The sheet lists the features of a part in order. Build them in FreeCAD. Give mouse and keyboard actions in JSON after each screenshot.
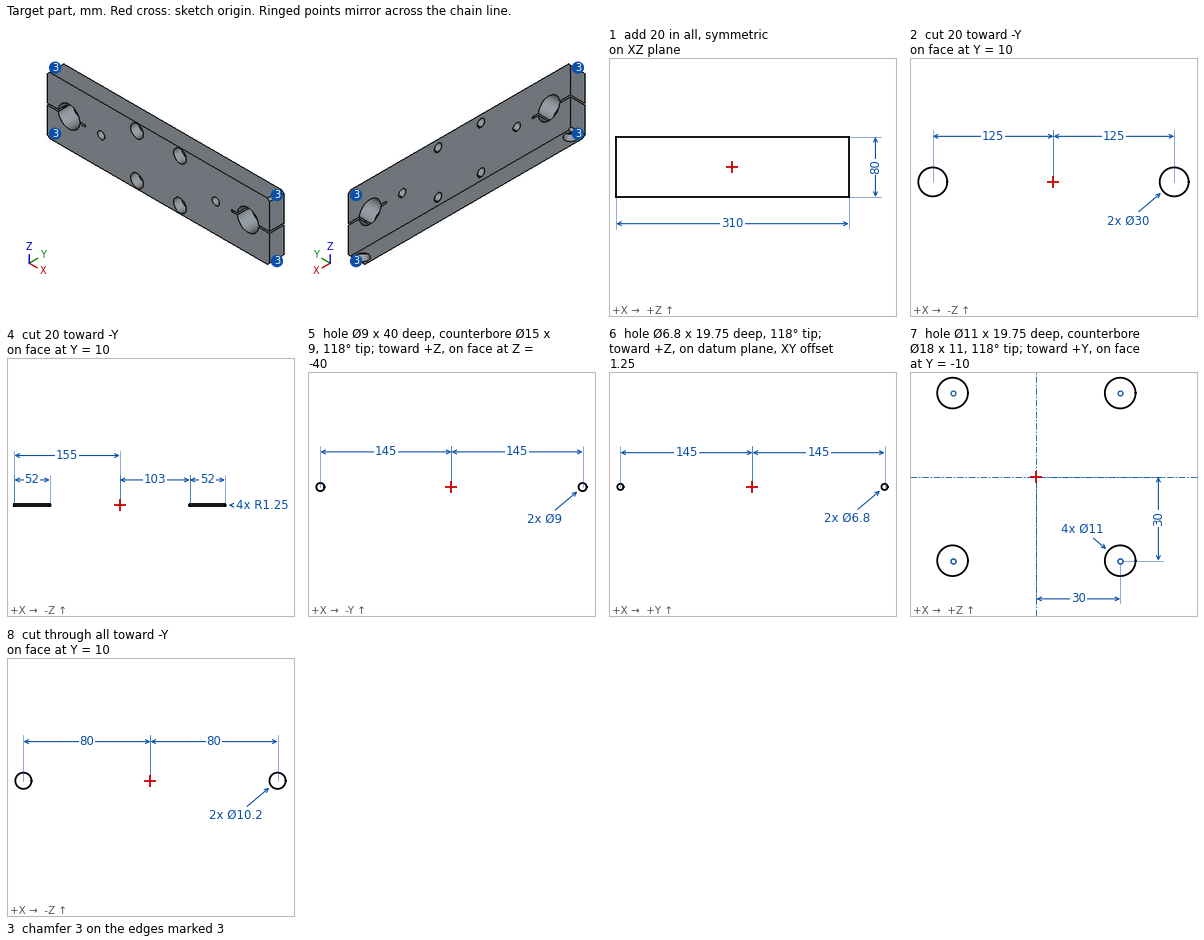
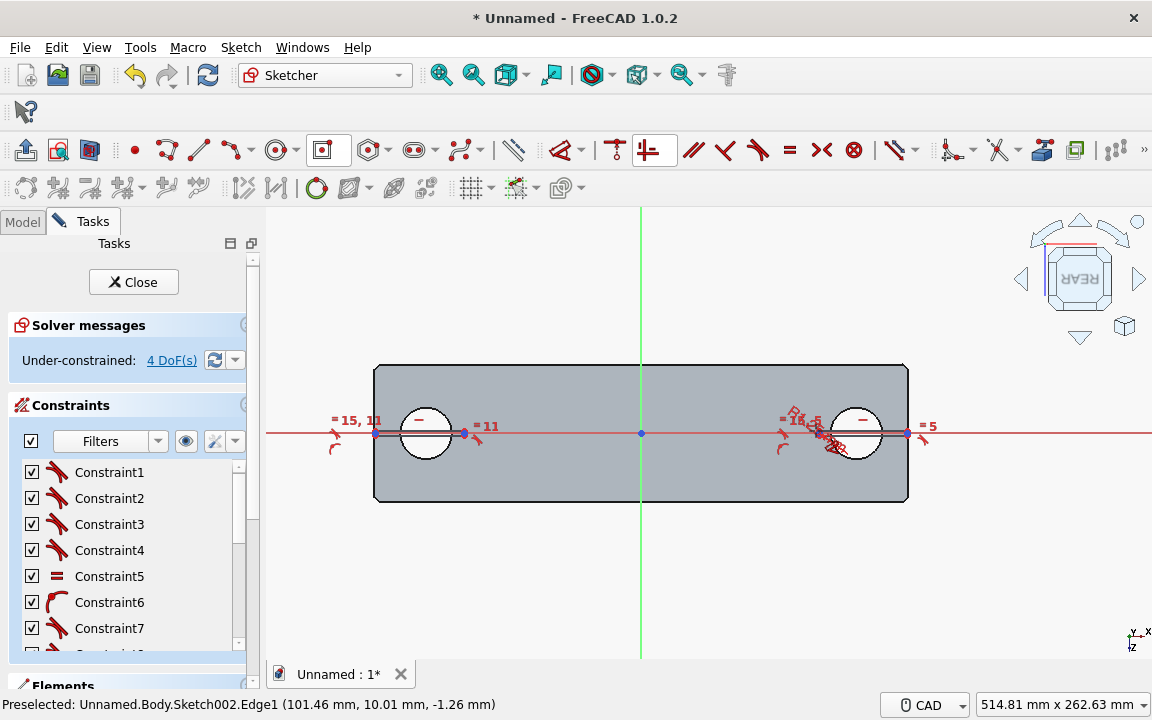
{"action": "scroll", "coordinate": [846, 431], "scroll_direction": "up", "scroll_amount": 10}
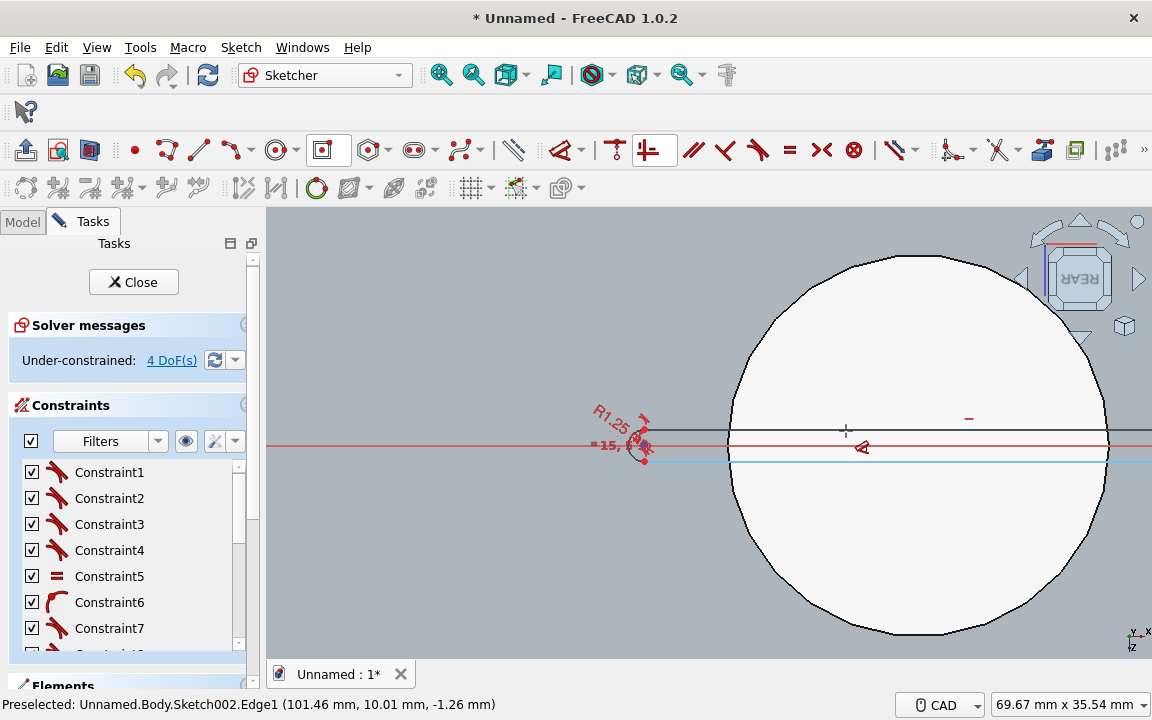
{"action": "left_click", "coordinate": [840, 430]}
{"action": "left_click", "coordinate": [816, 396]}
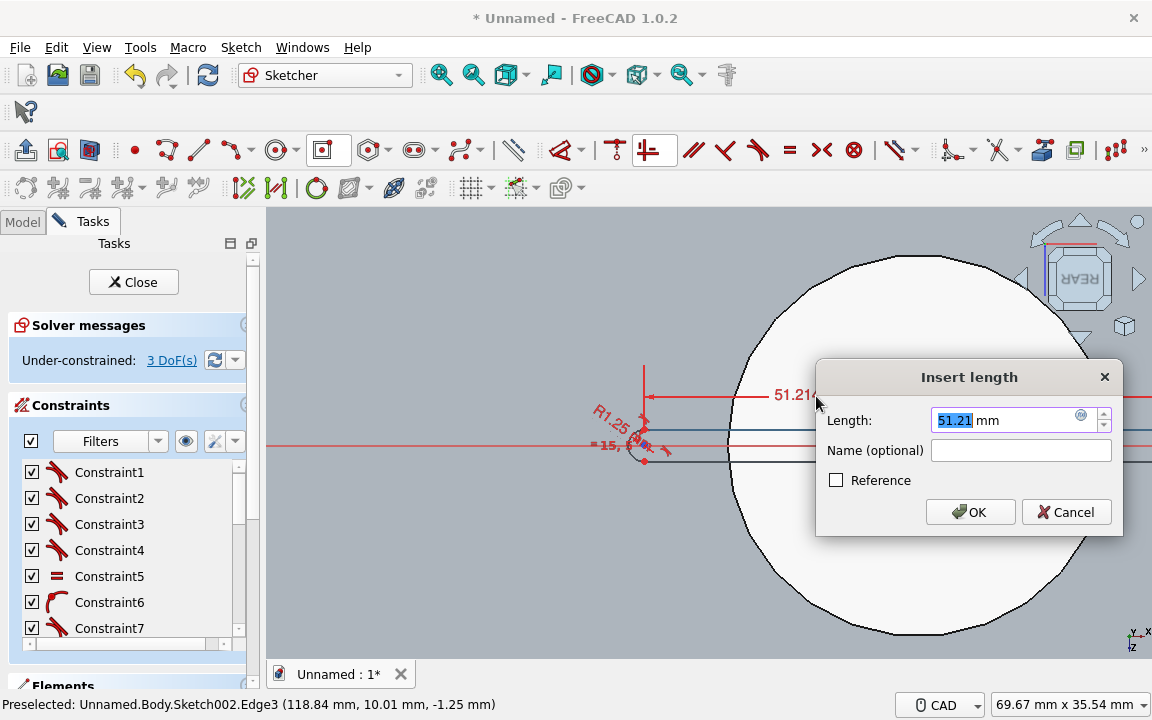
{"action": "type", "text": "52"}
{"action": "key", "text": "Return"}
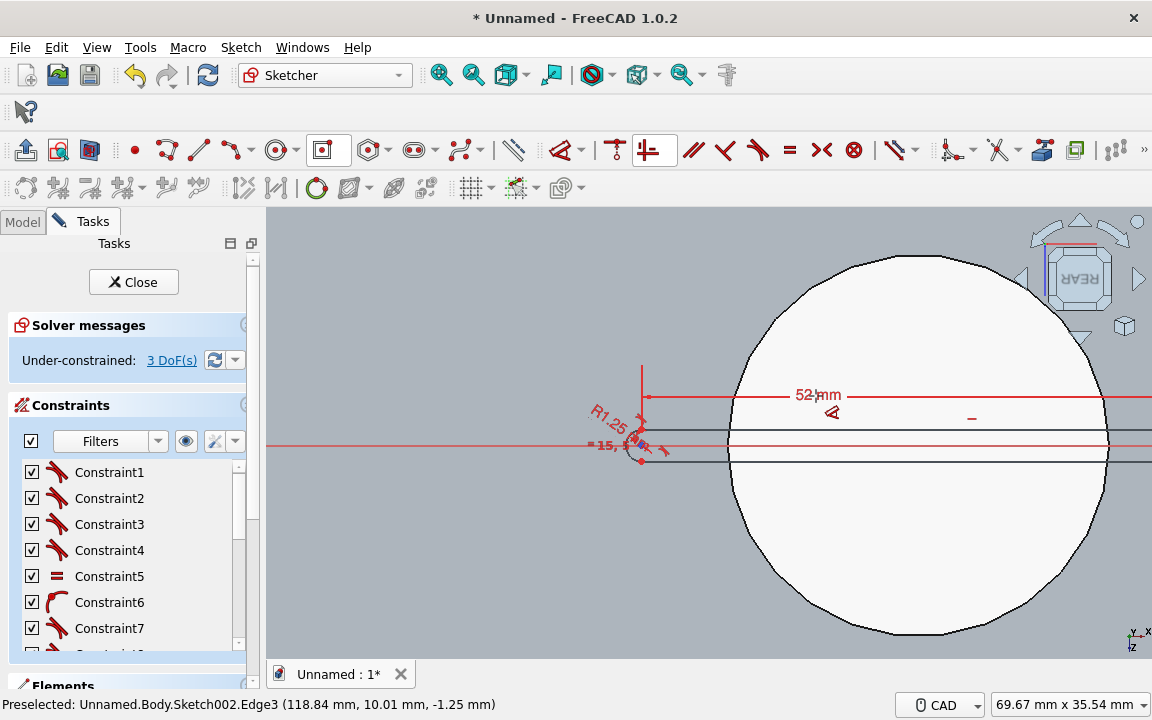
{"action": "scroll", "coordinate": [846, 431], "scroll_direction": "down", "scroll_amount": 10}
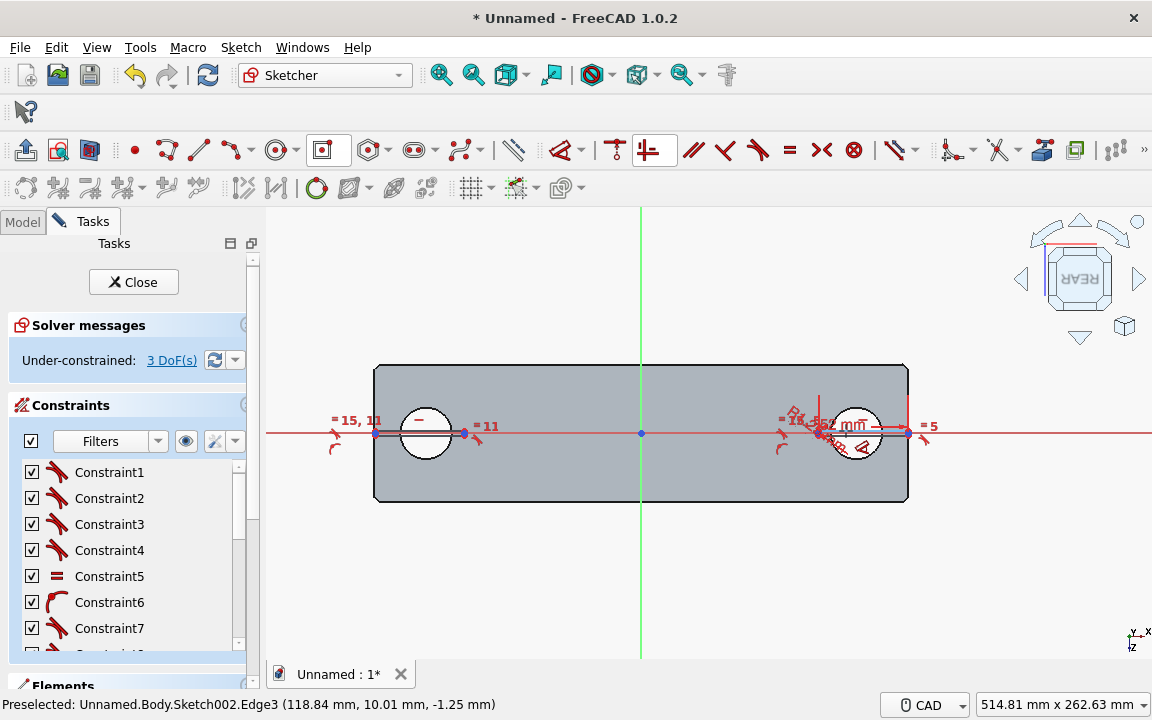
{"action": "scroll", "coordinate": [402, 431], "scroll_direction": "up", "scroll_amount": 10}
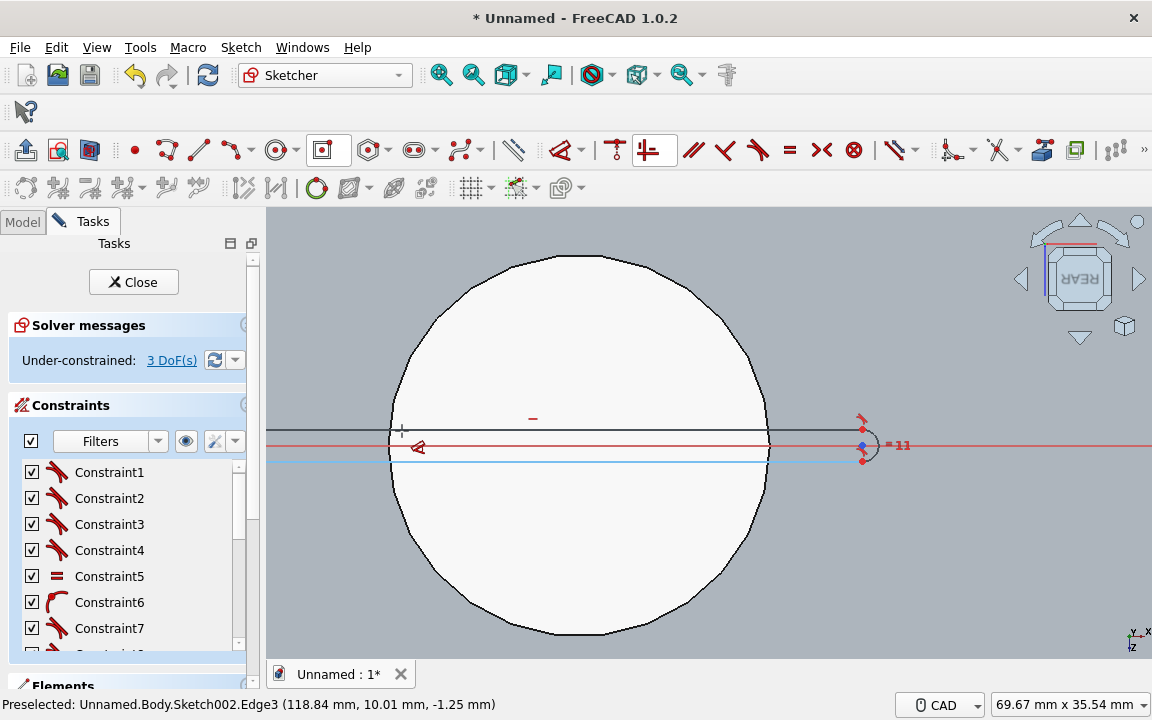
{"action": "left_click", "coordinate": [402, 430]}
{"action": "left_click", "coordinate": [578, 396]}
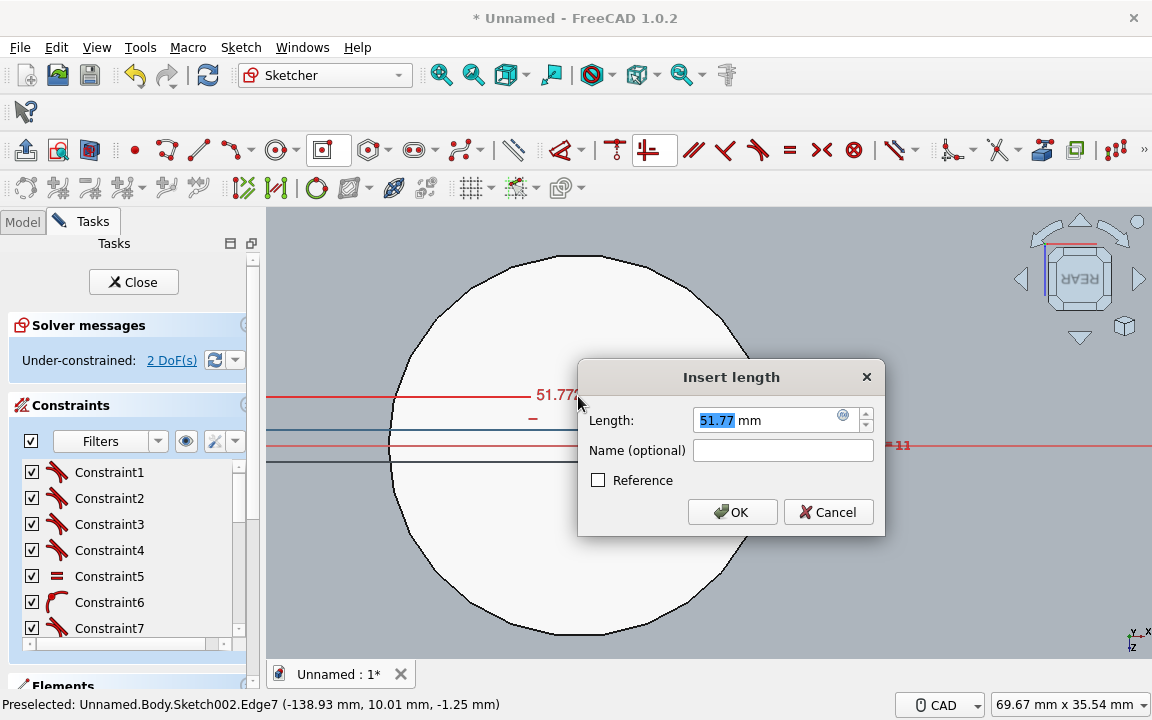
{"action": "type", "text": "52"}
{"action": "key", "text": "Return"}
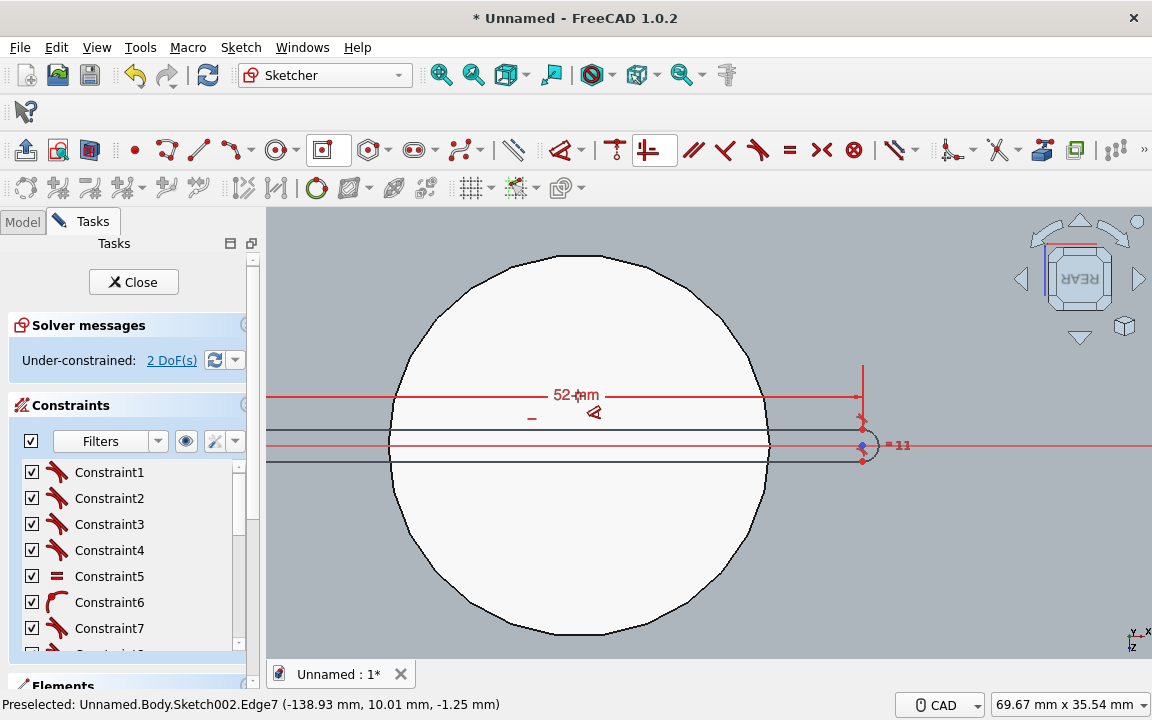
{"action": "scroll", "coordinate": [401, 431], "scroll_direction": "down", "scroll_amount": 10}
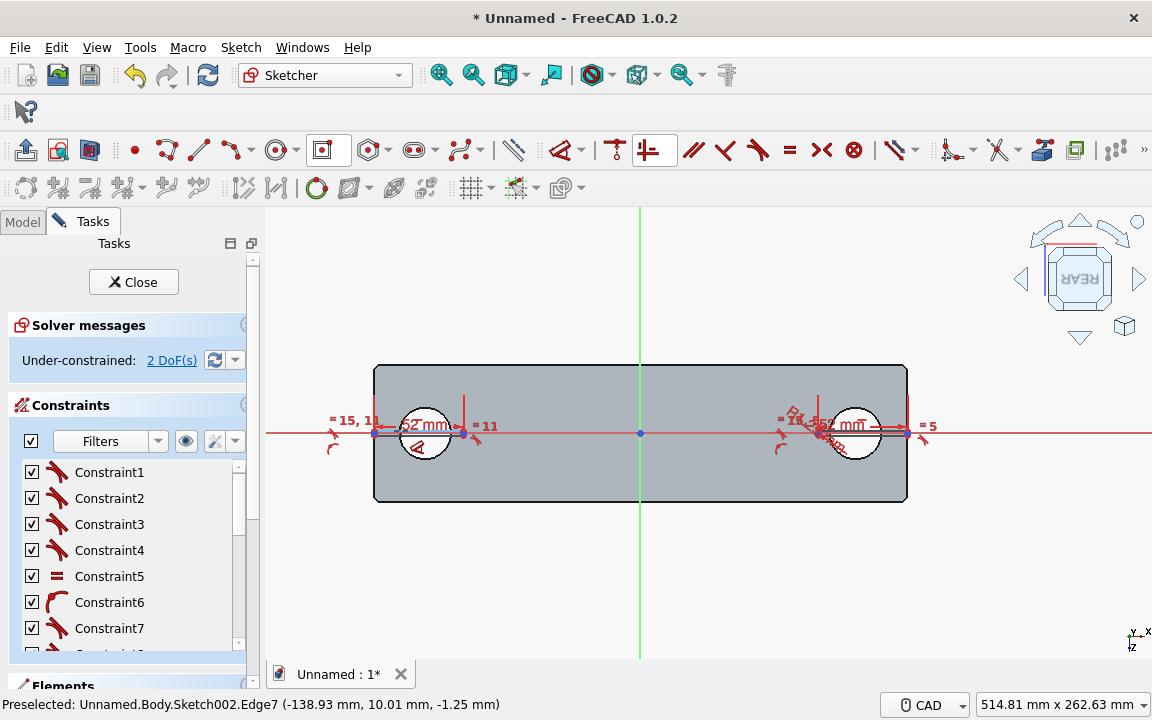
{"action": "scroll", "coordinate": [818, 431], "scroll_direction": "up", "scroll_amount": 9}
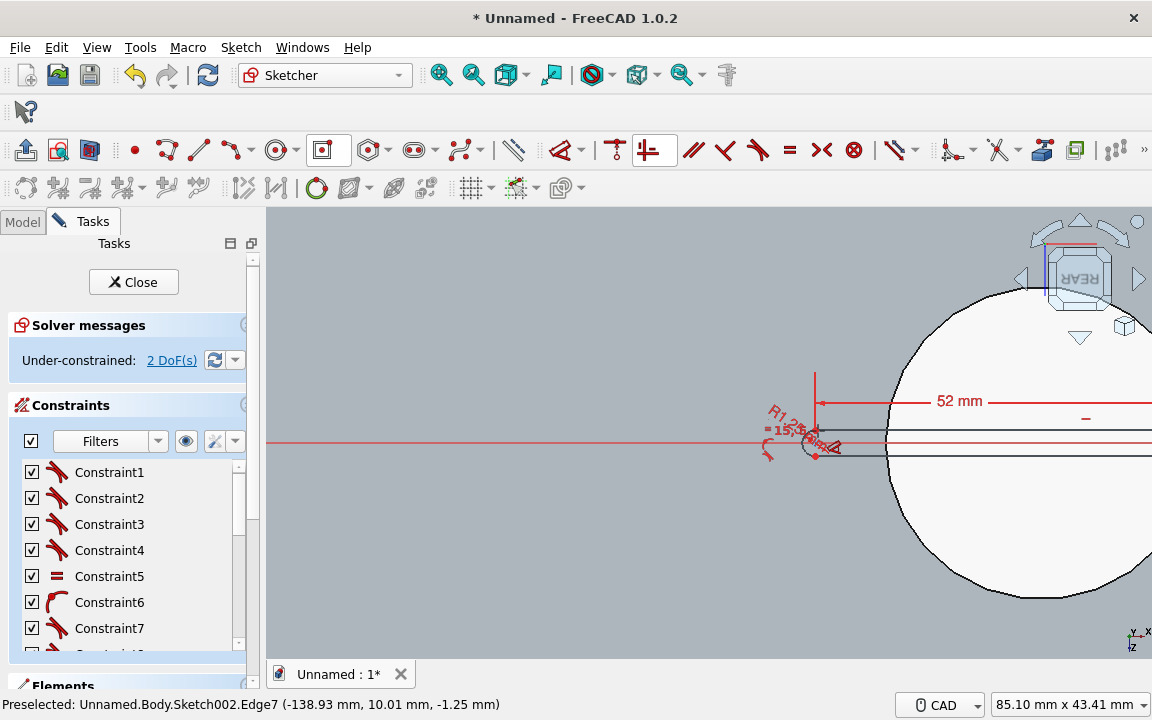
{"action": "left_click", "coordinate": [815, 430]}
{"action": "left_click", "coordinate": [555, 396]}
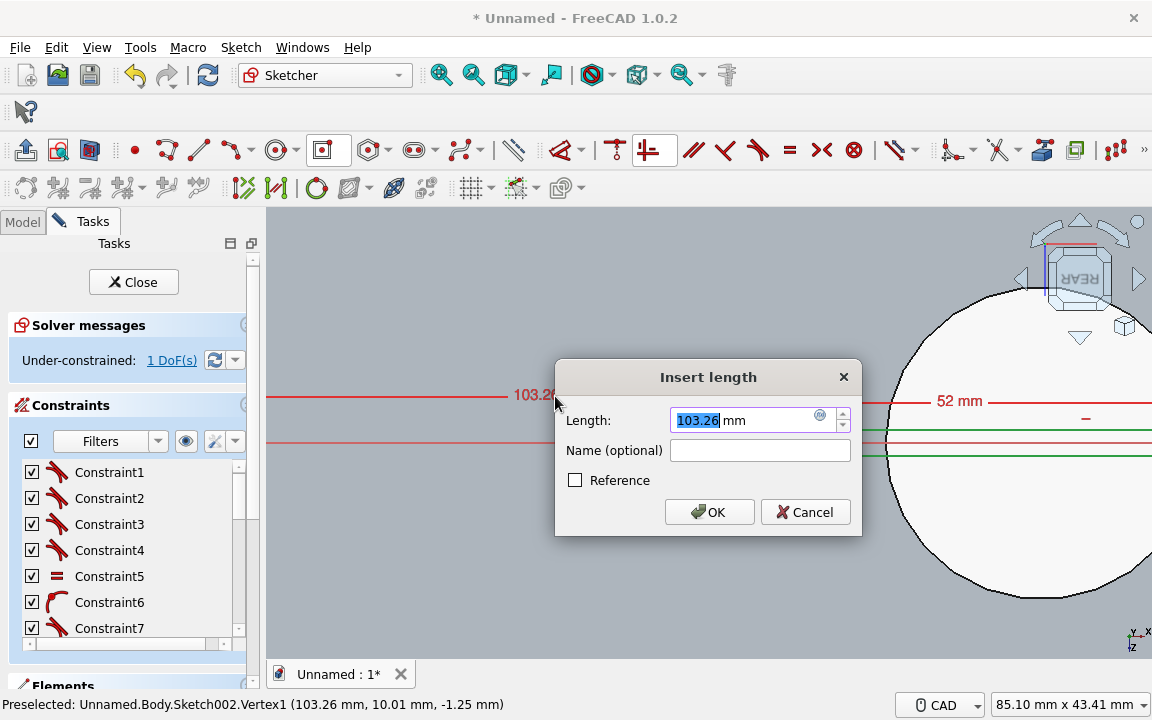
{"action": "type", "text": "103"}
{"action": "key", "text": "Return"}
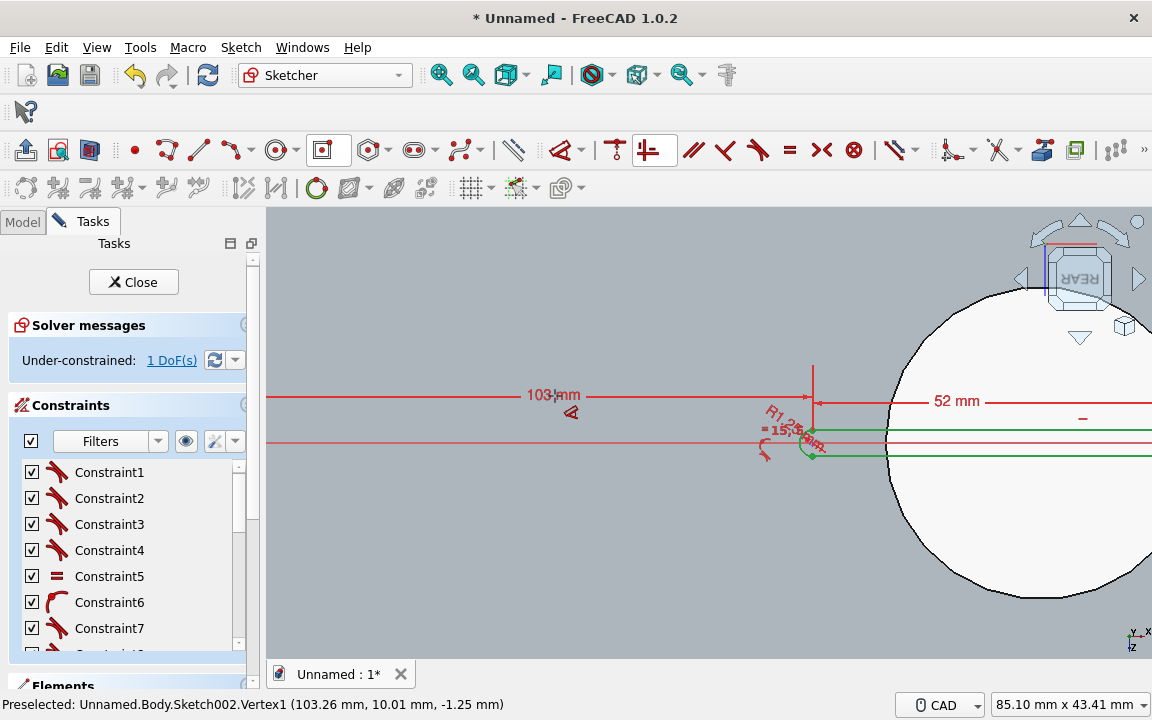
{"action": "scroll", "coordinate": [819, 431], "scroll_direction": "down", "scroll_amount": 9}